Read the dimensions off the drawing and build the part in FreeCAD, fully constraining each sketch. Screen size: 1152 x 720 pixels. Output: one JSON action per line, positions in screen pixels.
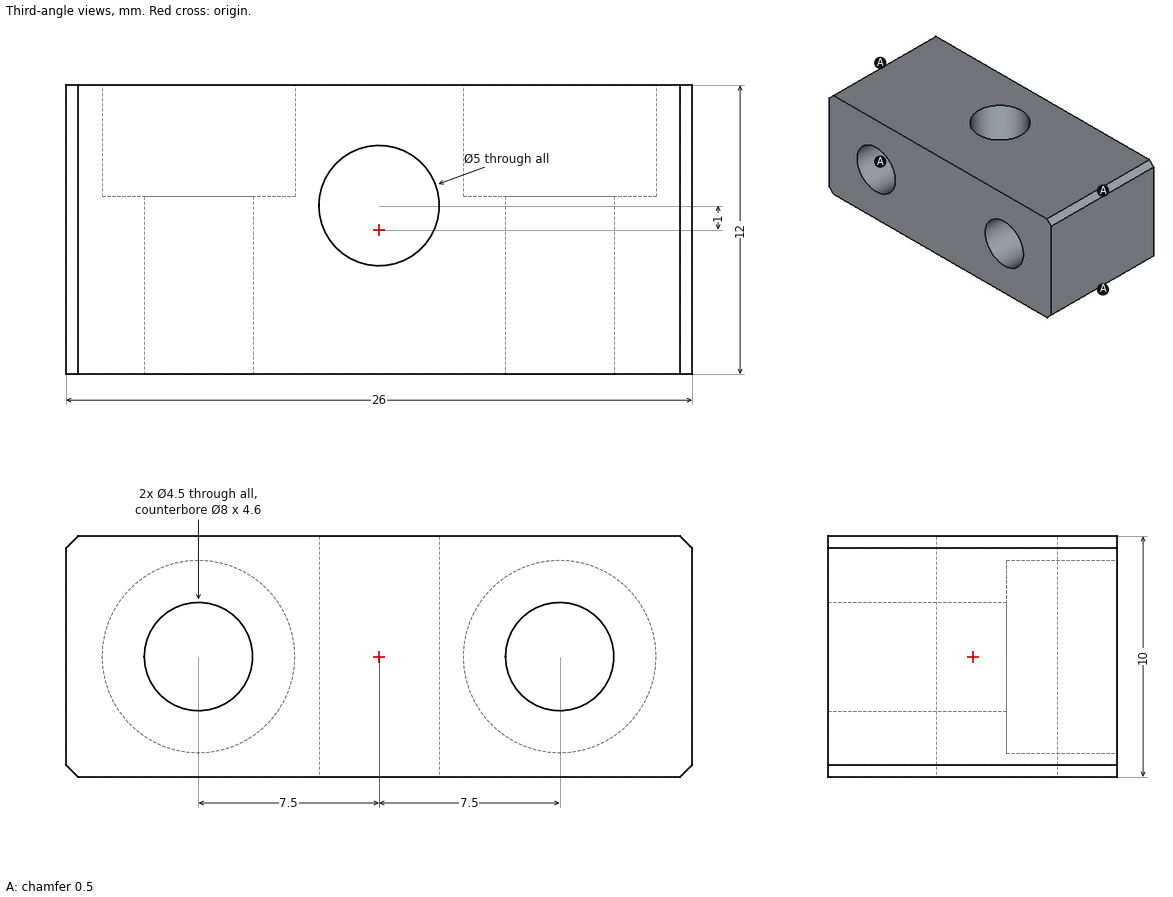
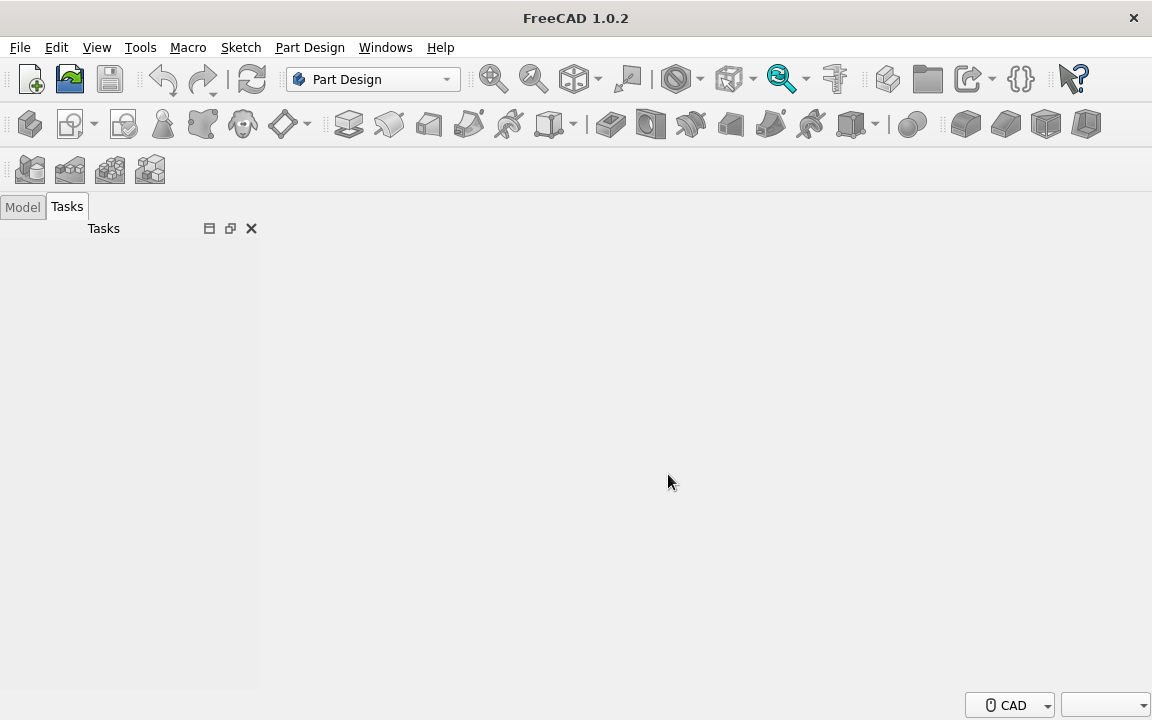
{"action": "key", "text": "ctrl+n"}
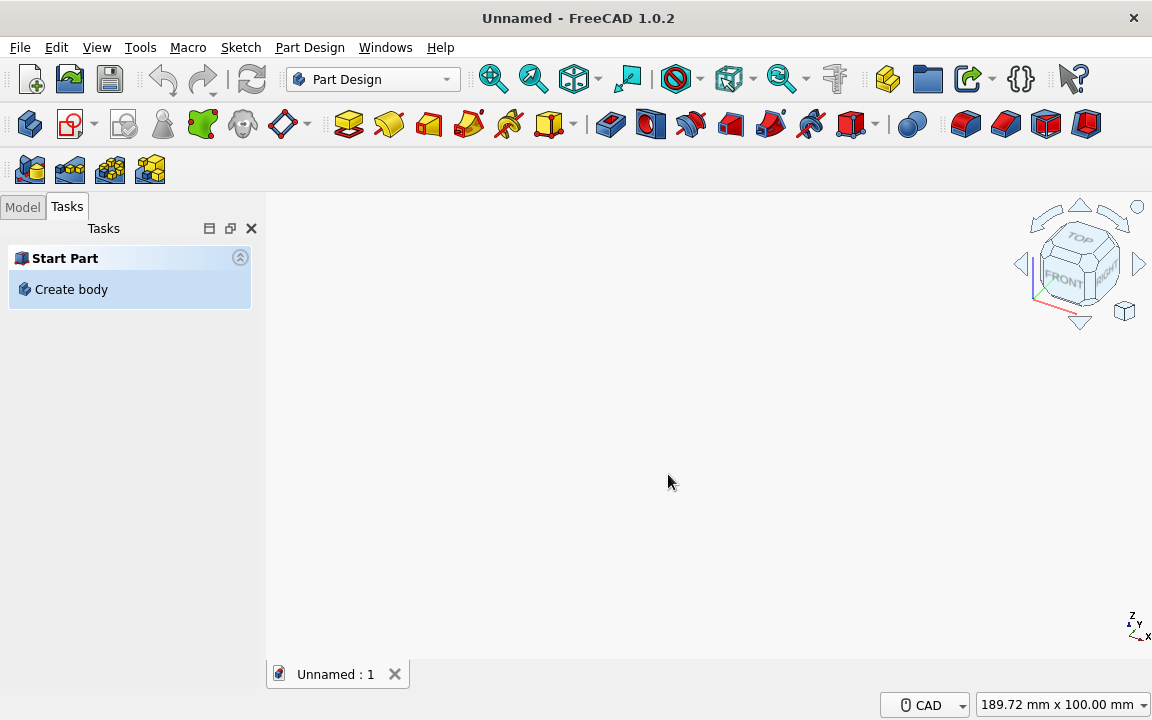
{"action": "left_click", "coordinate": [70, 124]}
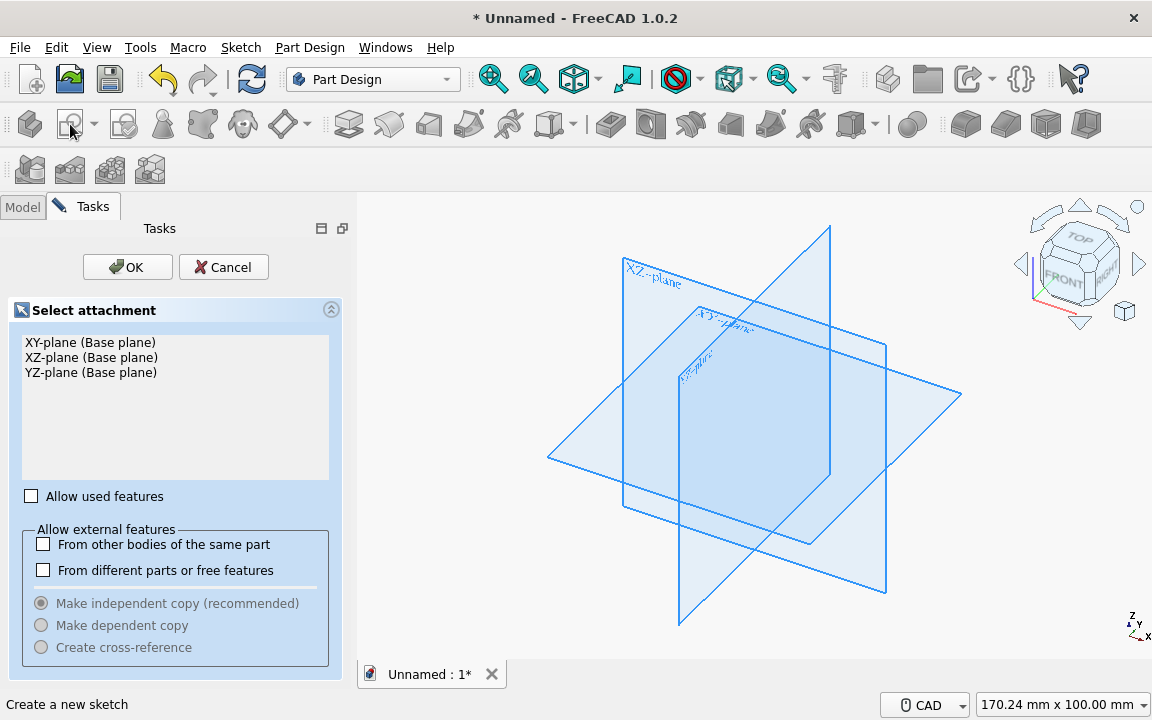
{"action": "left_click", "coordinate": [82, 342]}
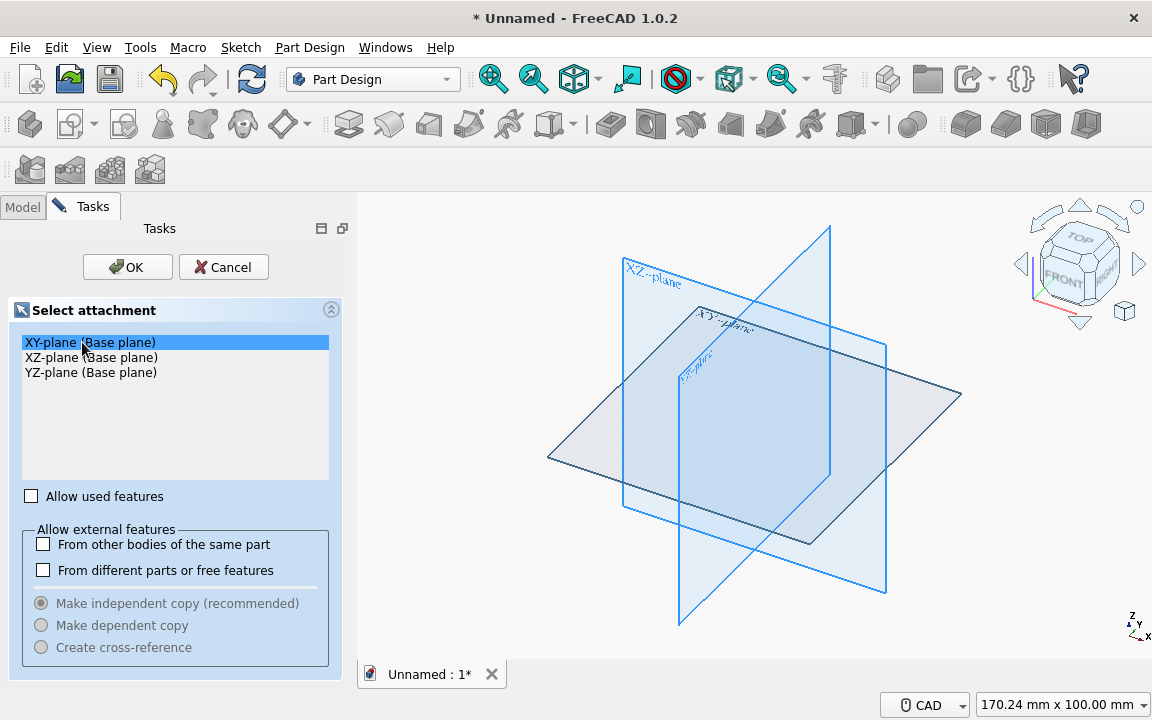
{"action": "left_click", "coordinate": [128, 267]}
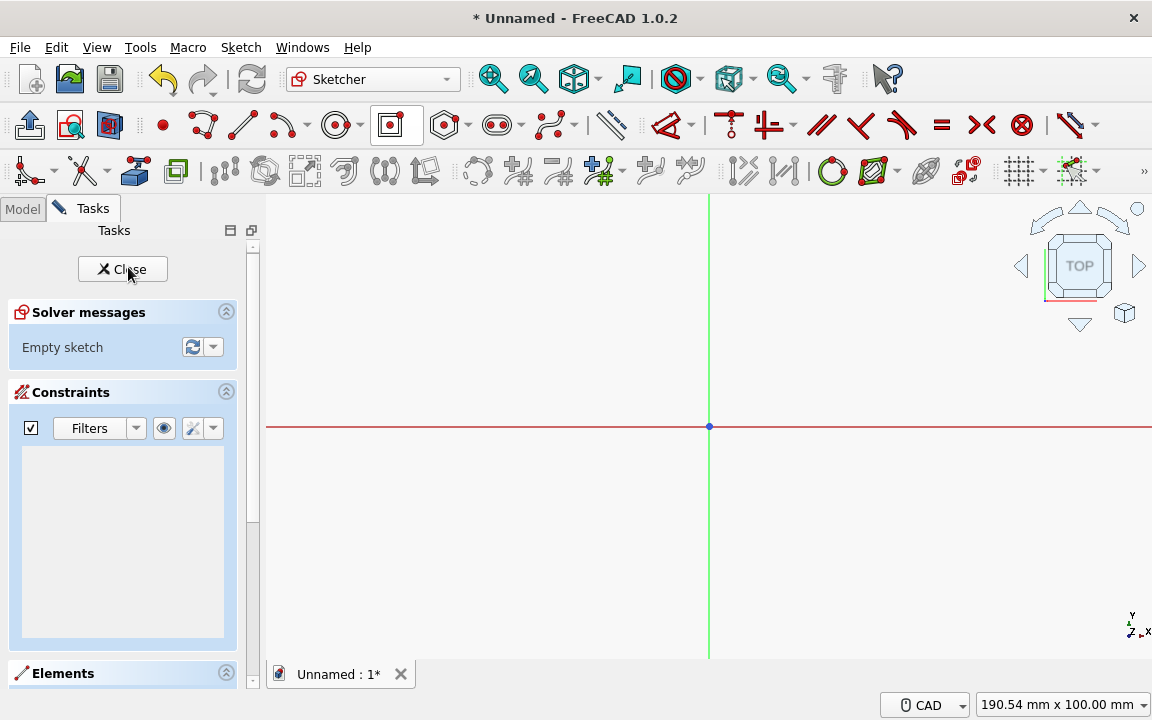
{"action": "scroll", "coordinate": [731, 426], "scroll_direction": "up", "scroll_amount": 7}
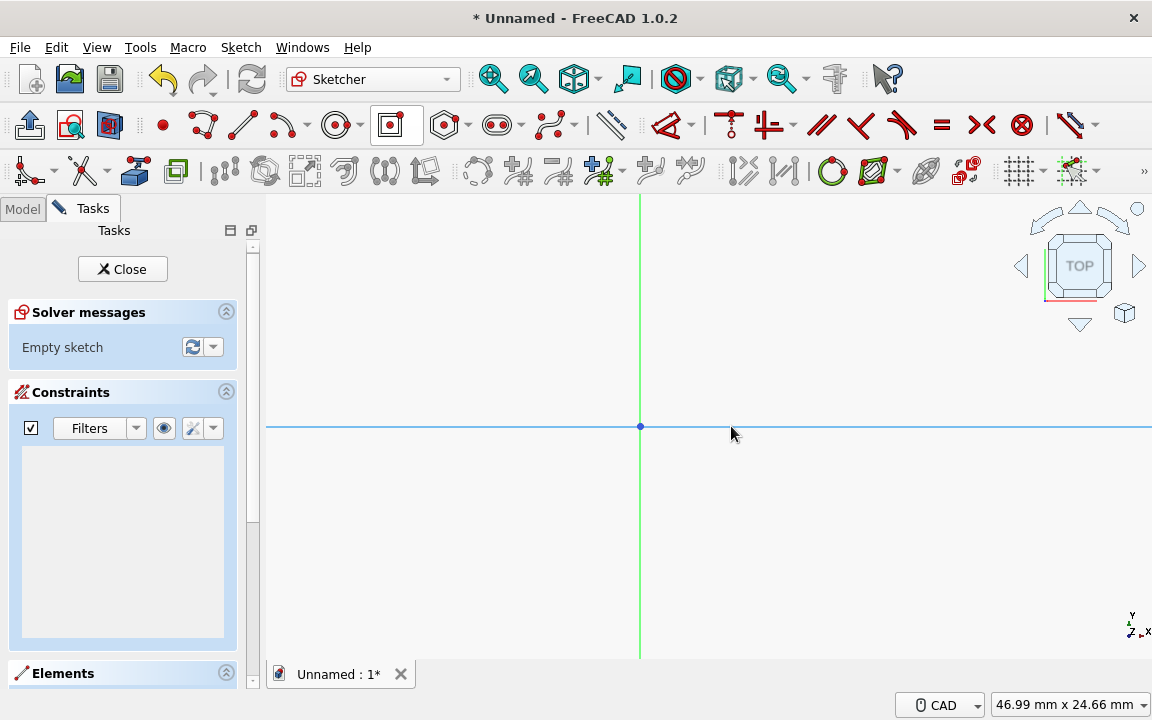
{"action": "key", "text": "g v"}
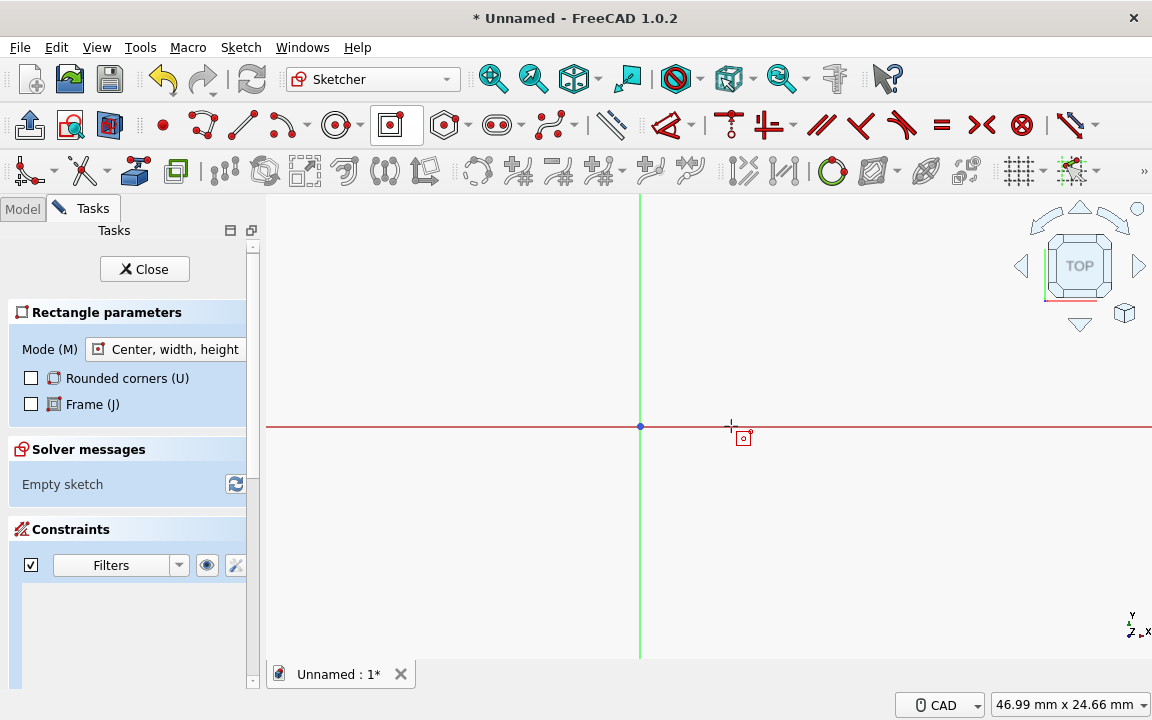
{"action": "left_click", "coordinate": [640, 426]}
{"action": "left_click", "coordinate": [885, 313]}
{"action": "key", "text": "Escape"}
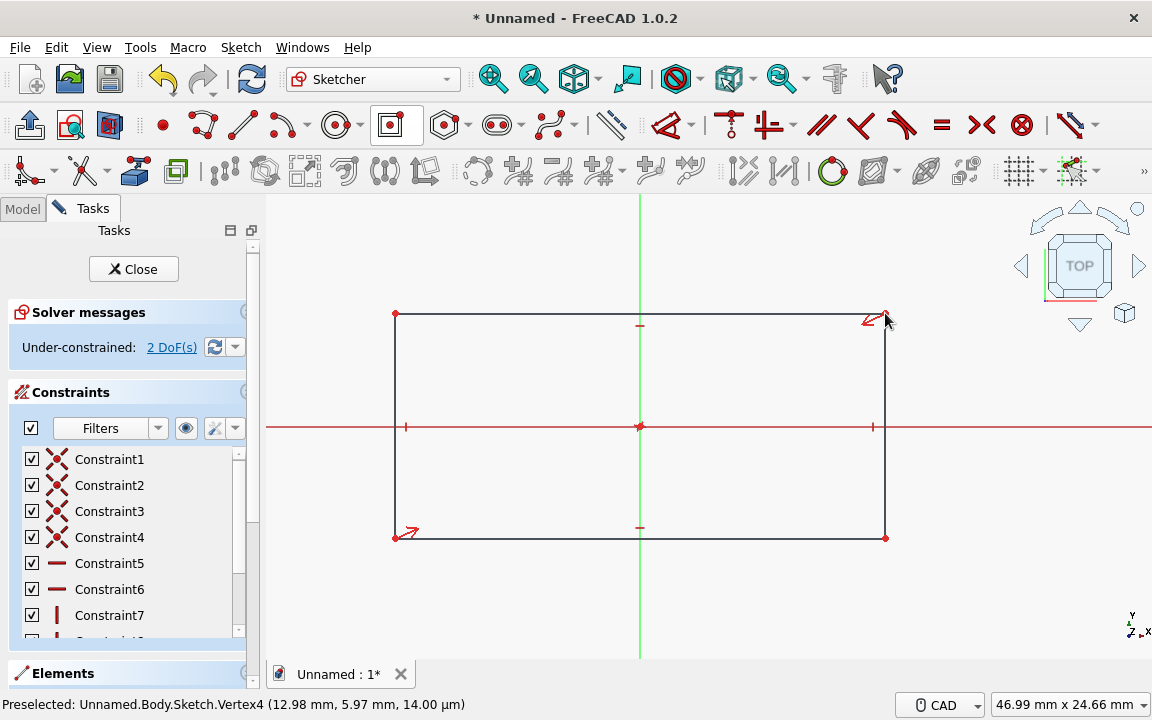
{"action": "left_click", "coordinate": [542, 539]}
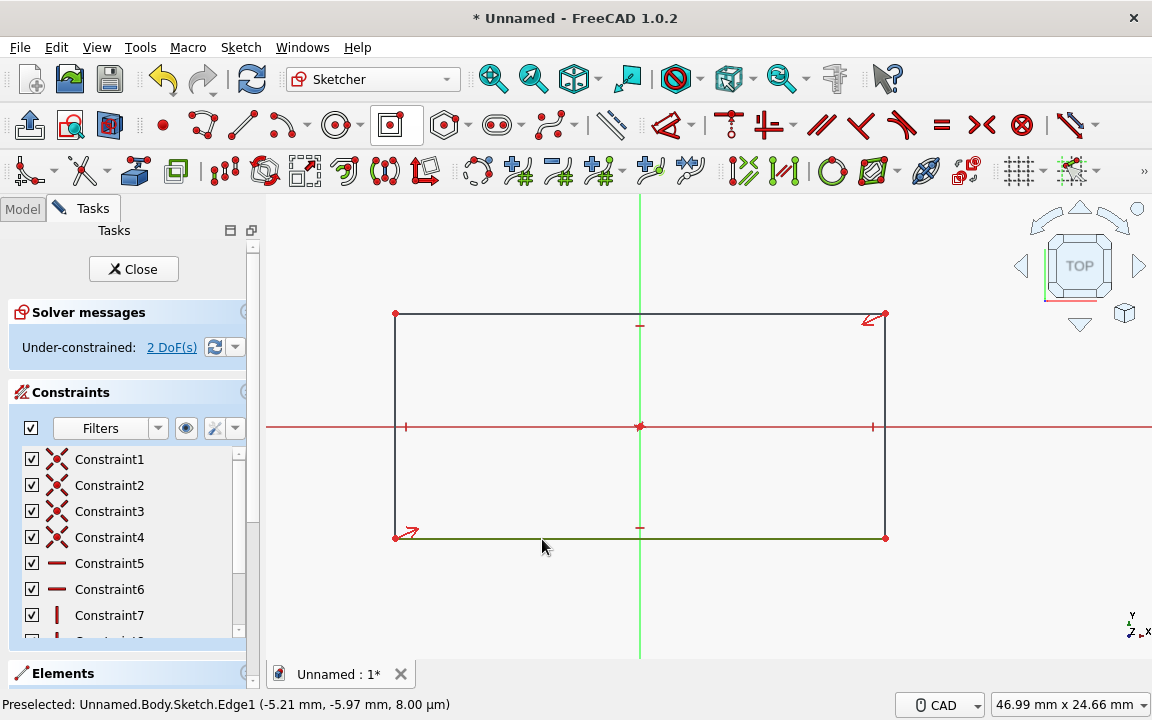
{"action": "key", "text": "l"}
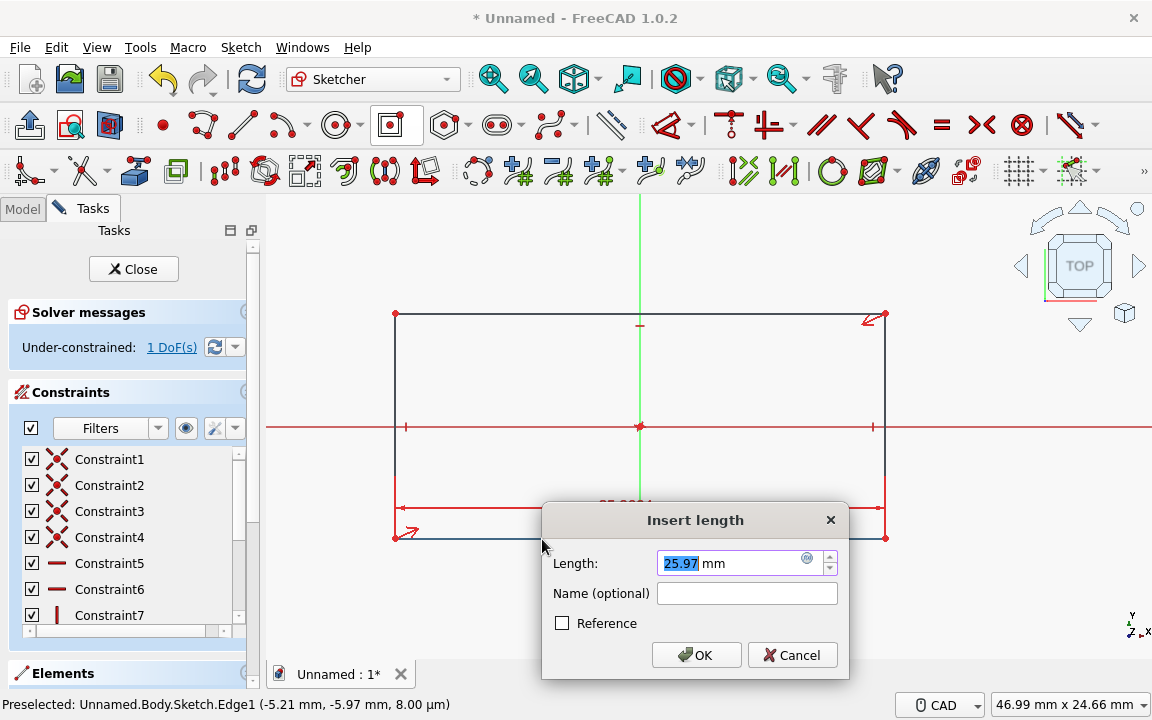
{"action": "type", "text": "26"}
{"action": "key", "text": "Return"}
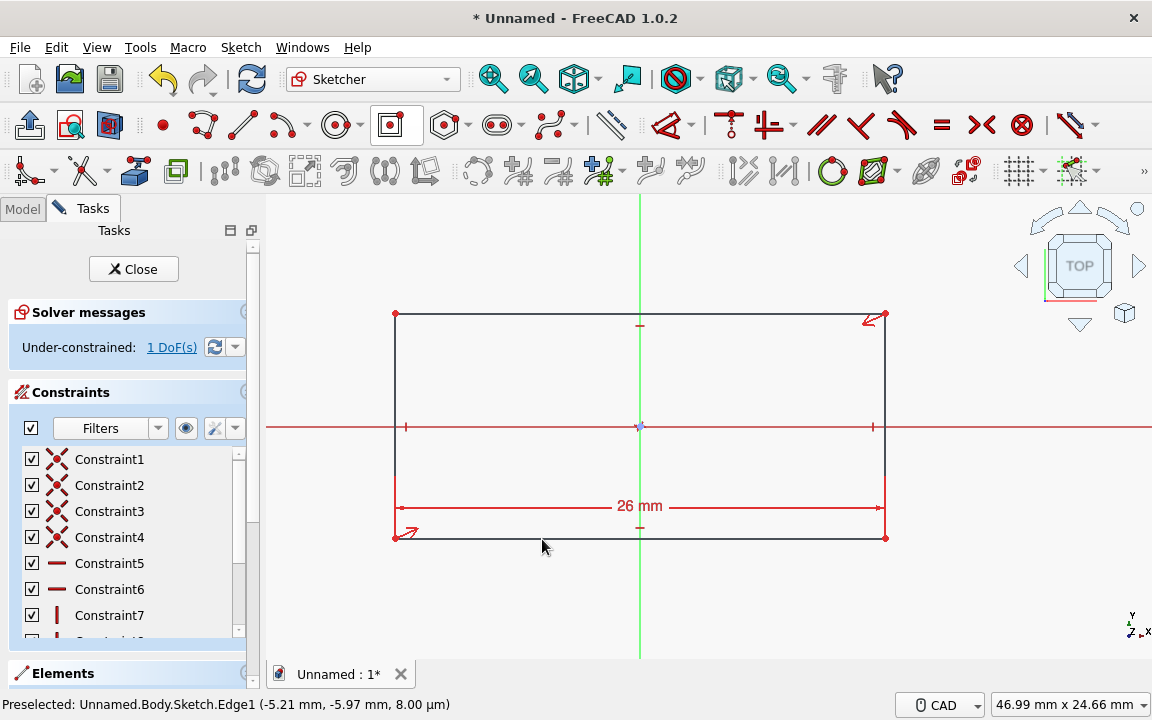
{"action": "left_click", "coordinate": [885, 472]}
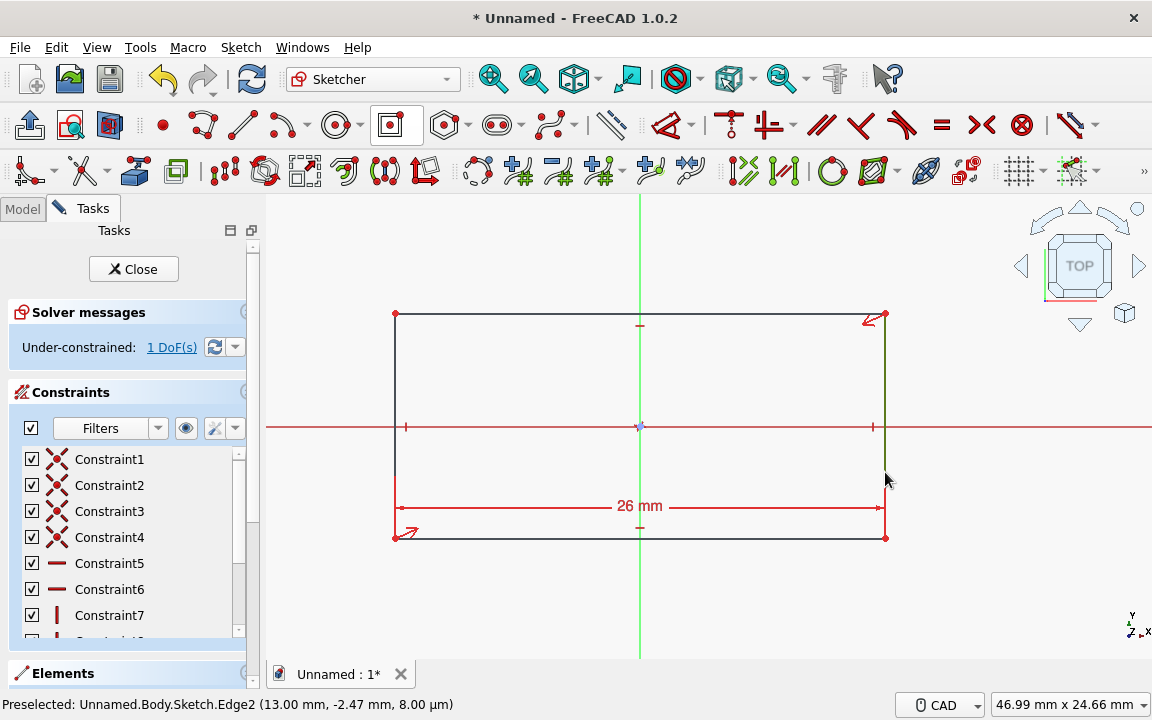
{"action": "key", "text": "i"}